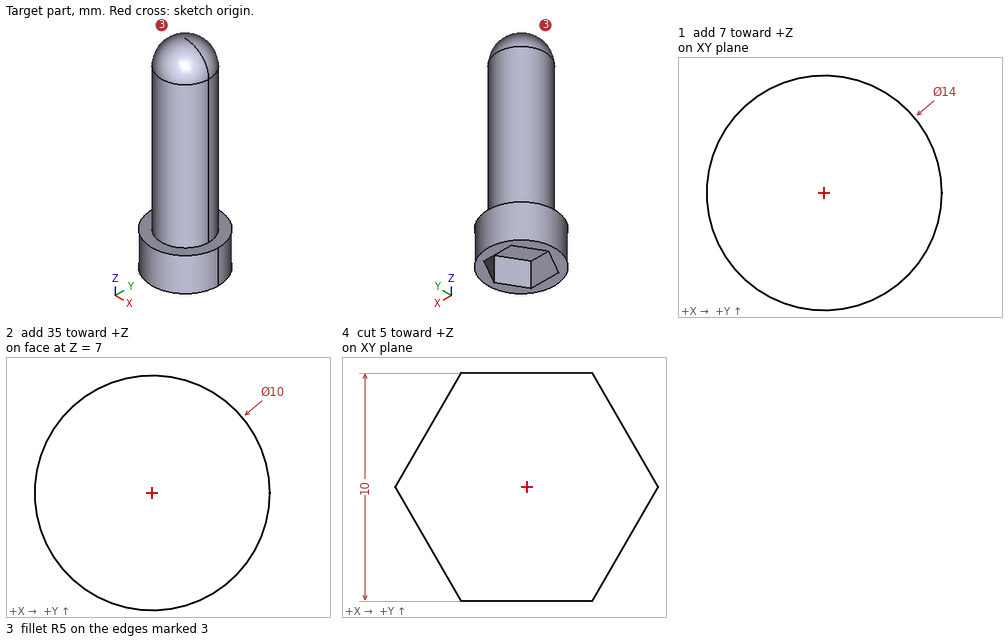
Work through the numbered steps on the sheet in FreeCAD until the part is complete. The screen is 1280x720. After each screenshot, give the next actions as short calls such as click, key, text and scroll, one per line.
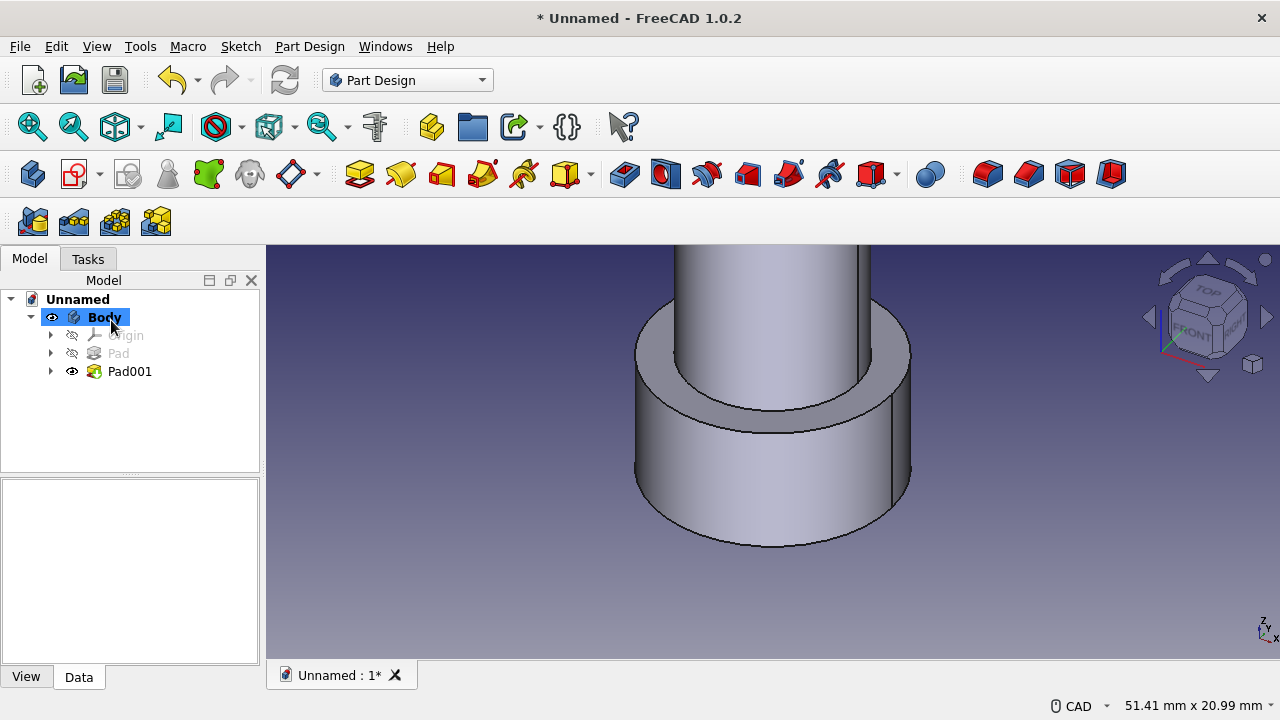
key(v)
key(f)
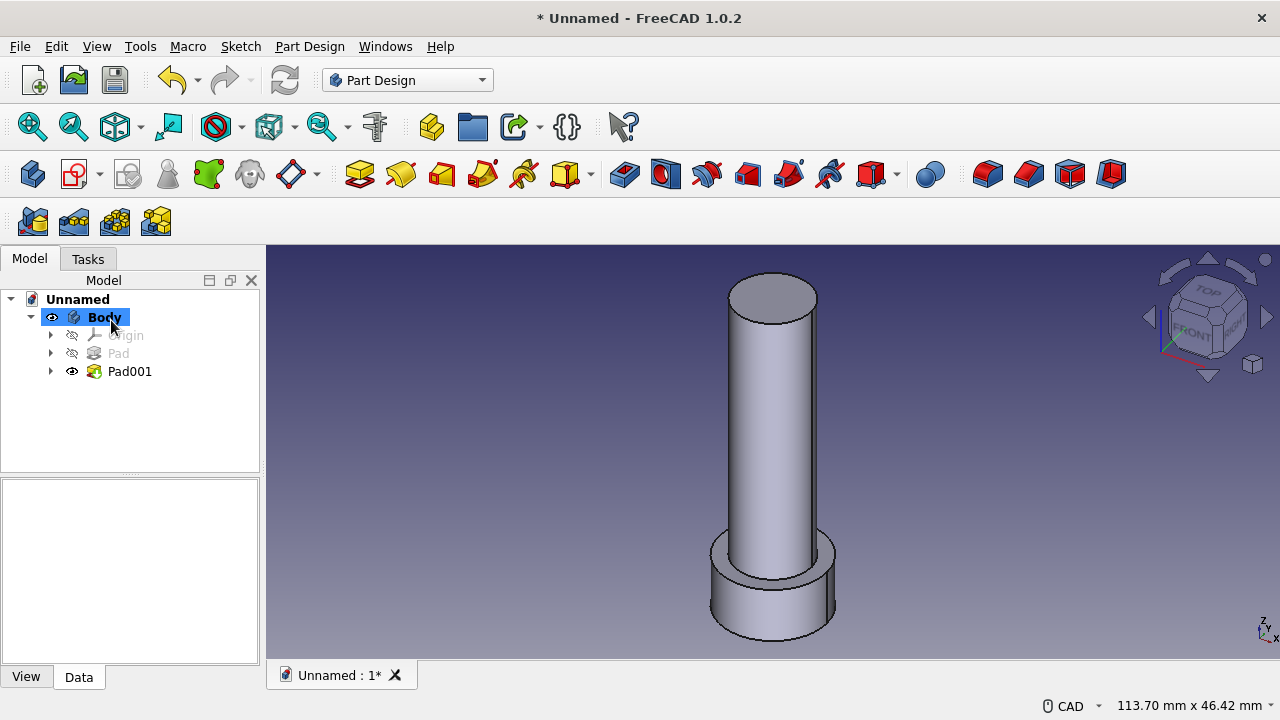
click(734, 285)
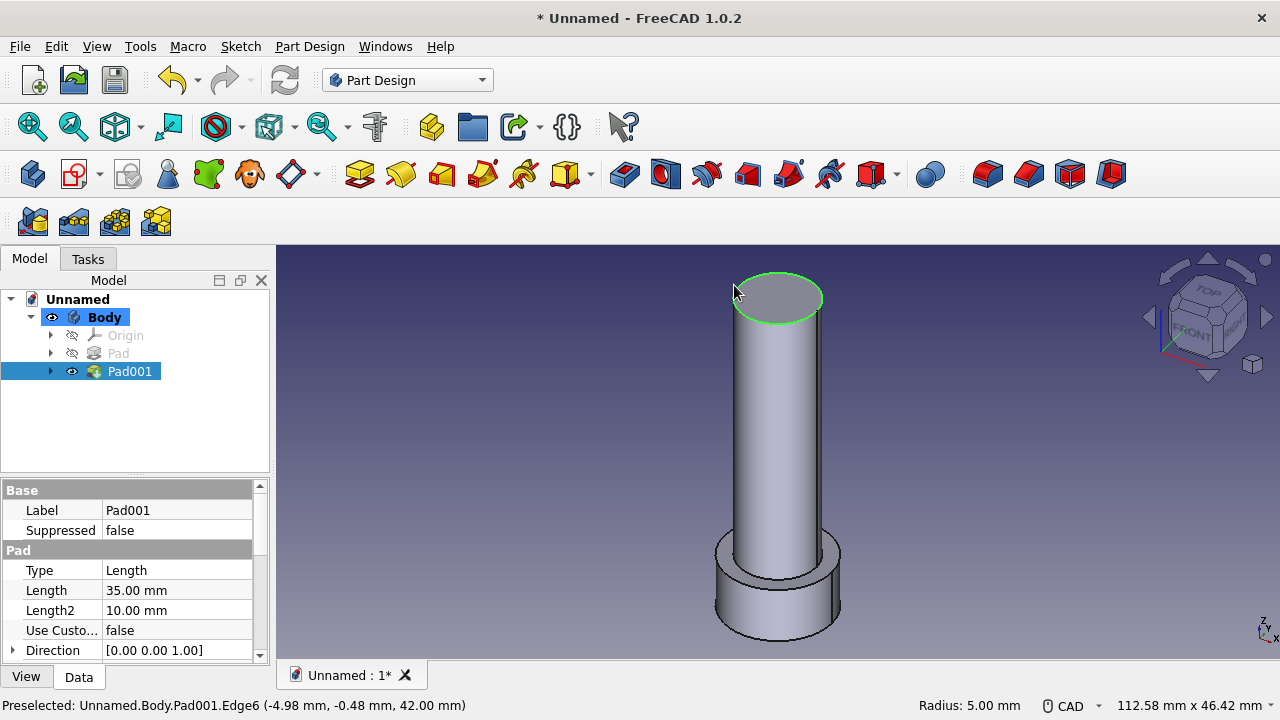
click(988, 174)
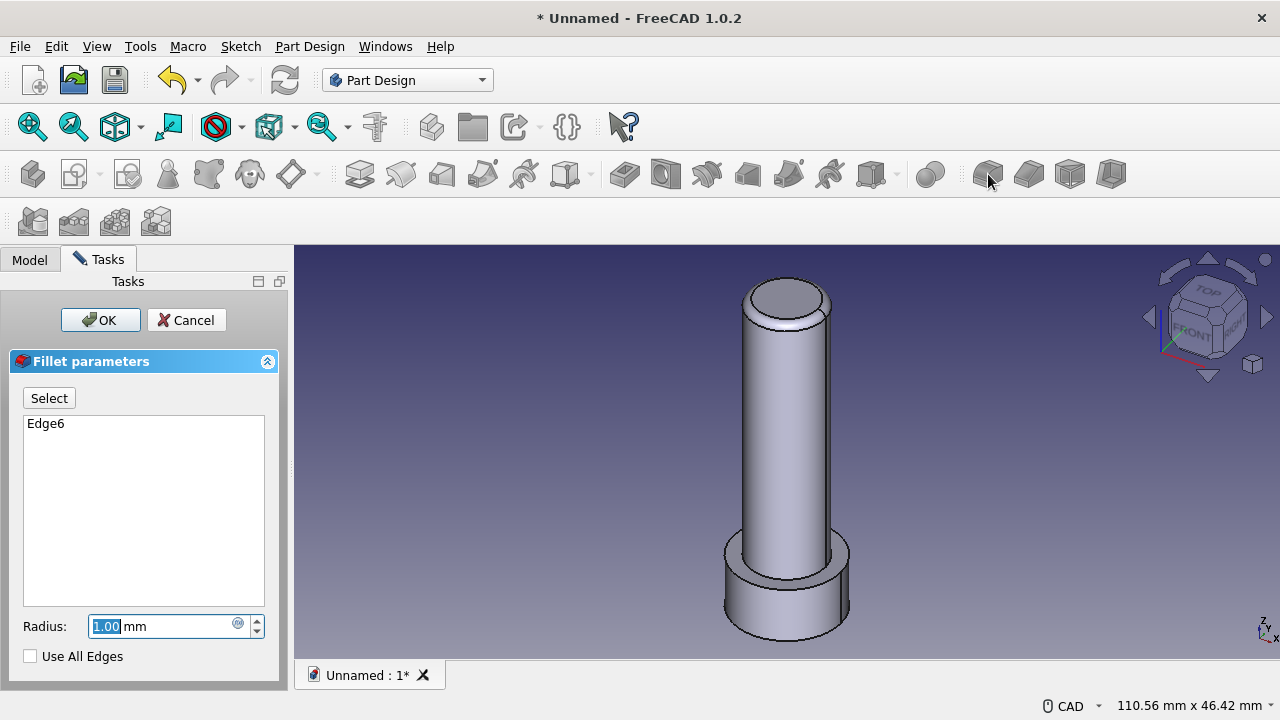
text(5)
key(Tab)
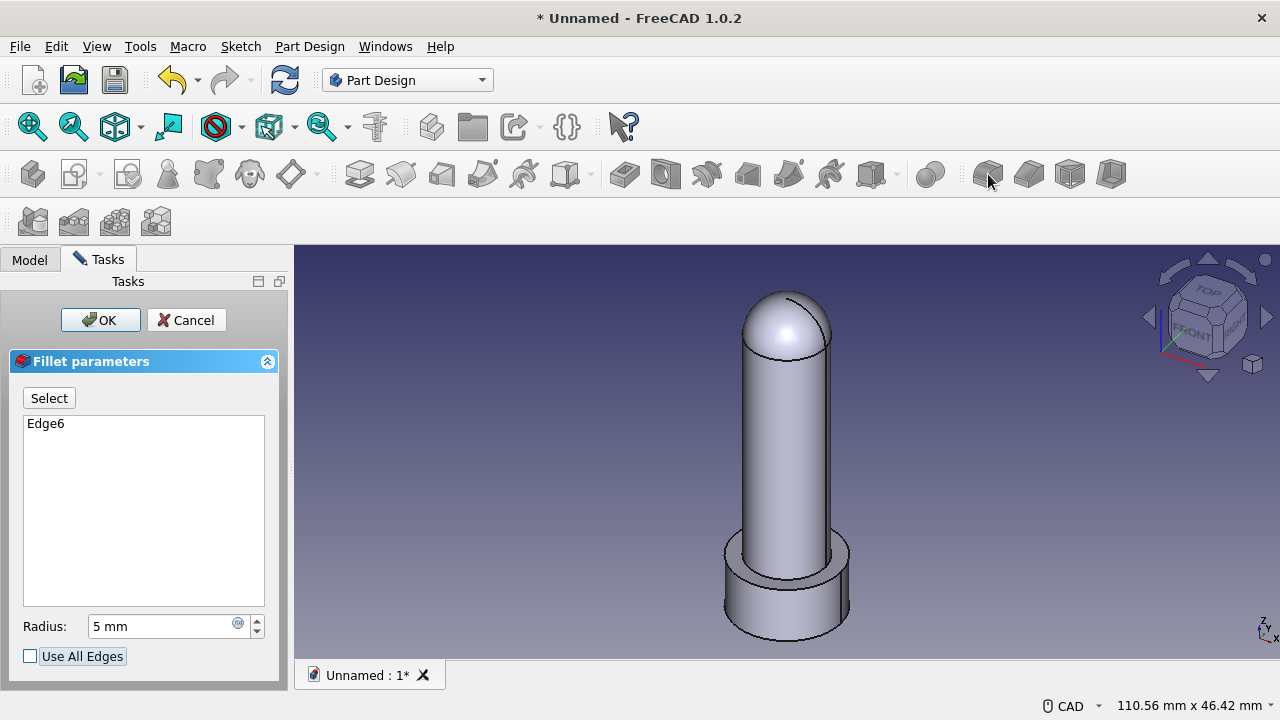
click(101, 320)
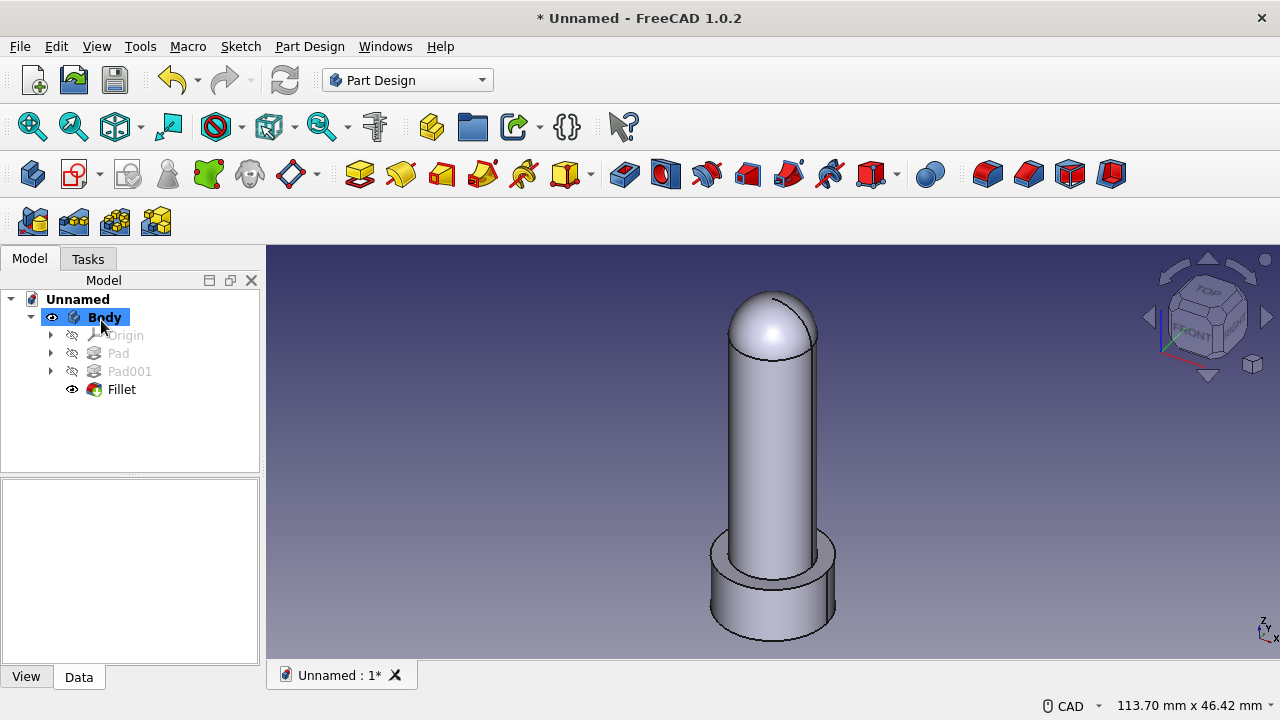
click(74, 174)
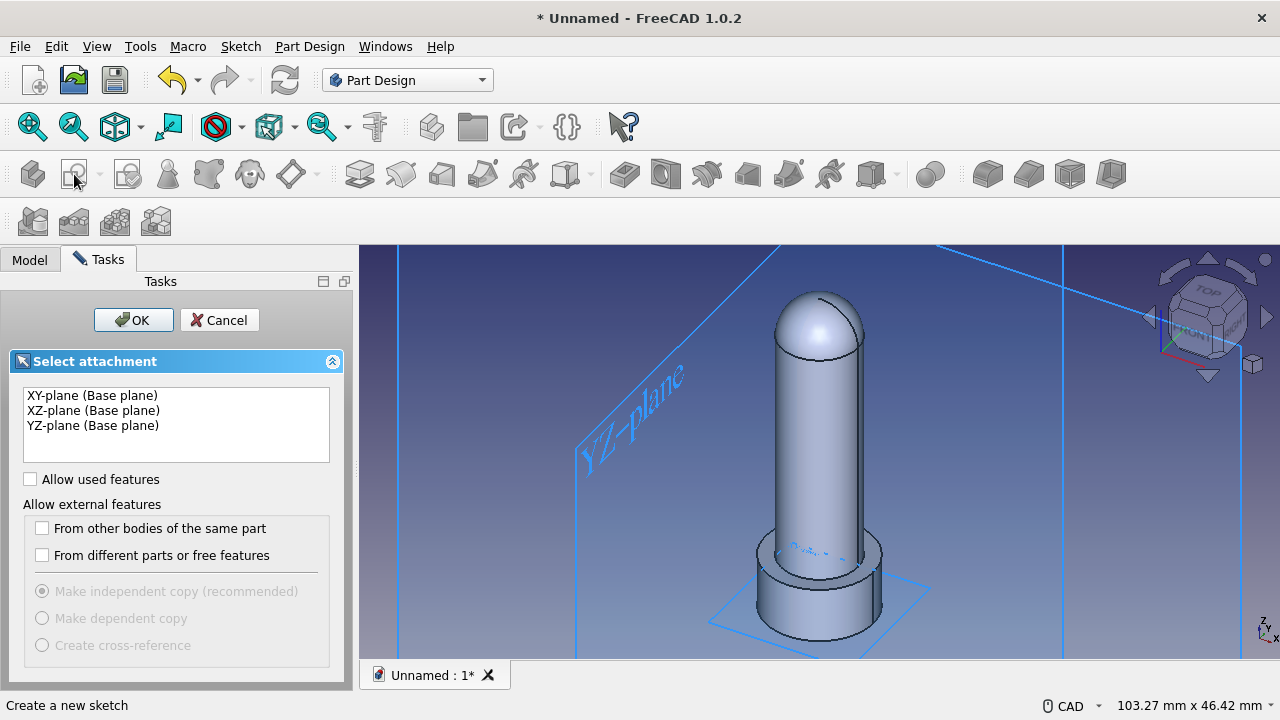
click(84, 396)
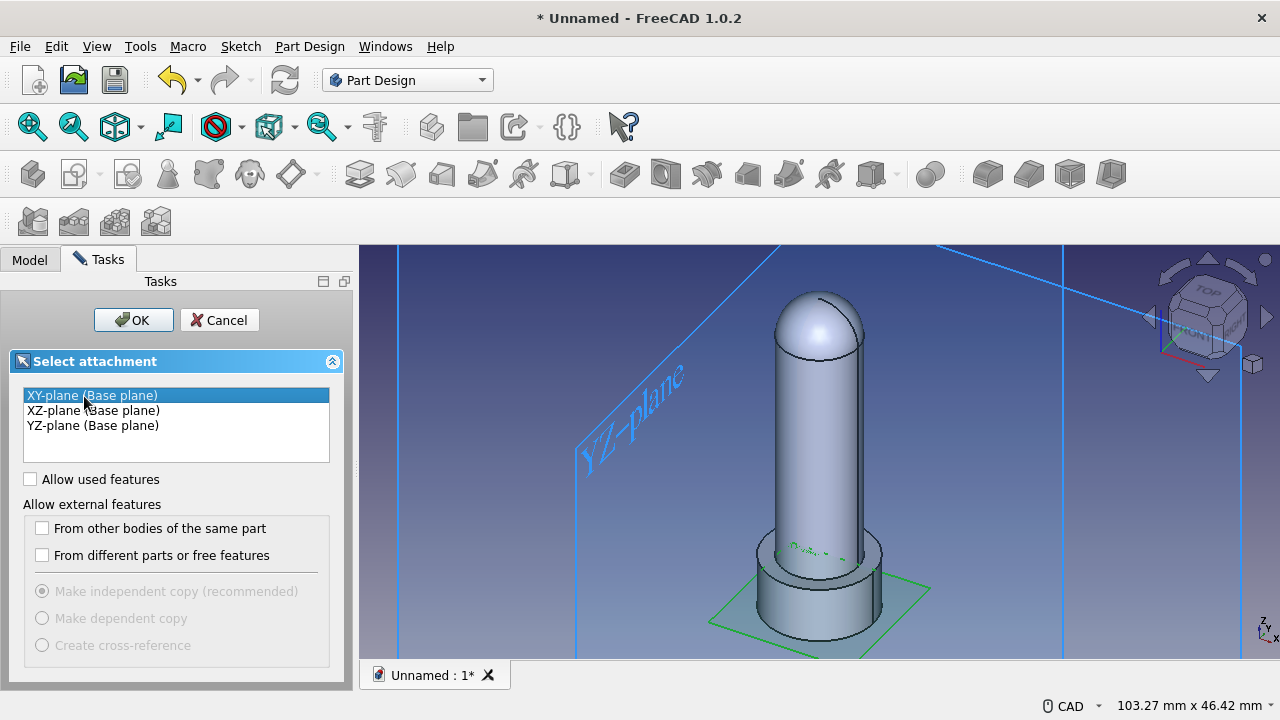
click(134, 320)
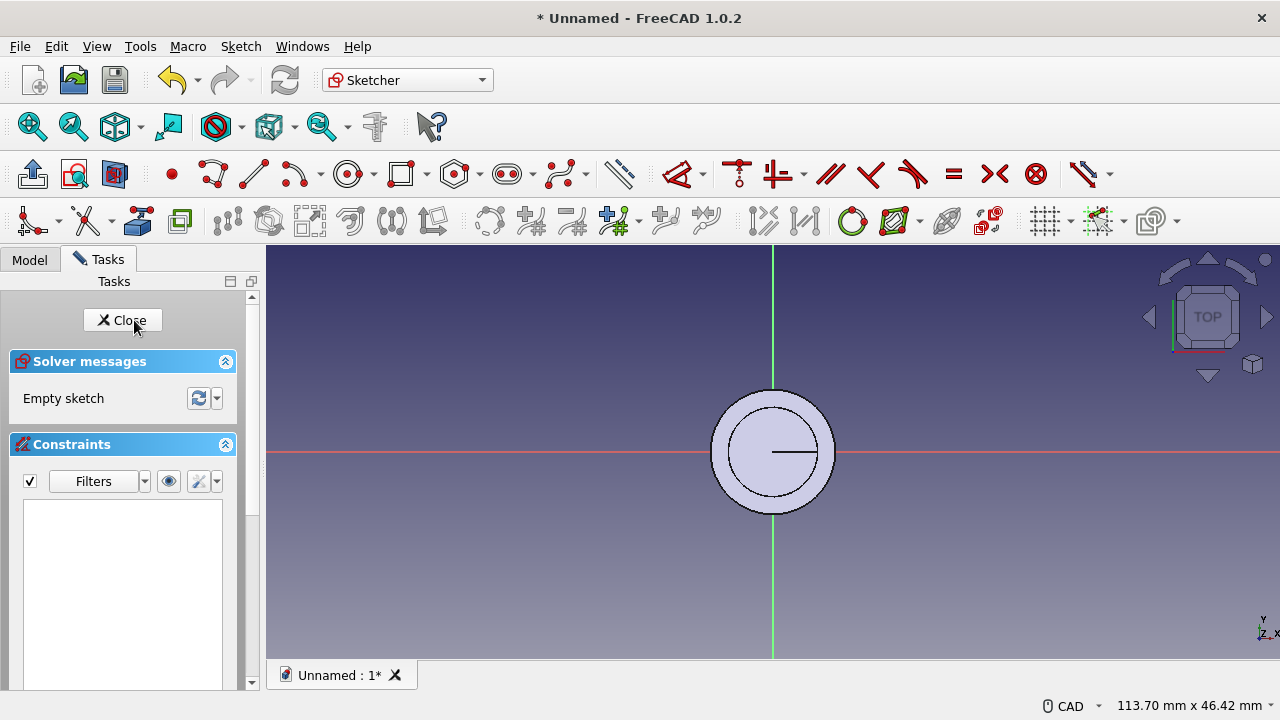
key(q)
key(s)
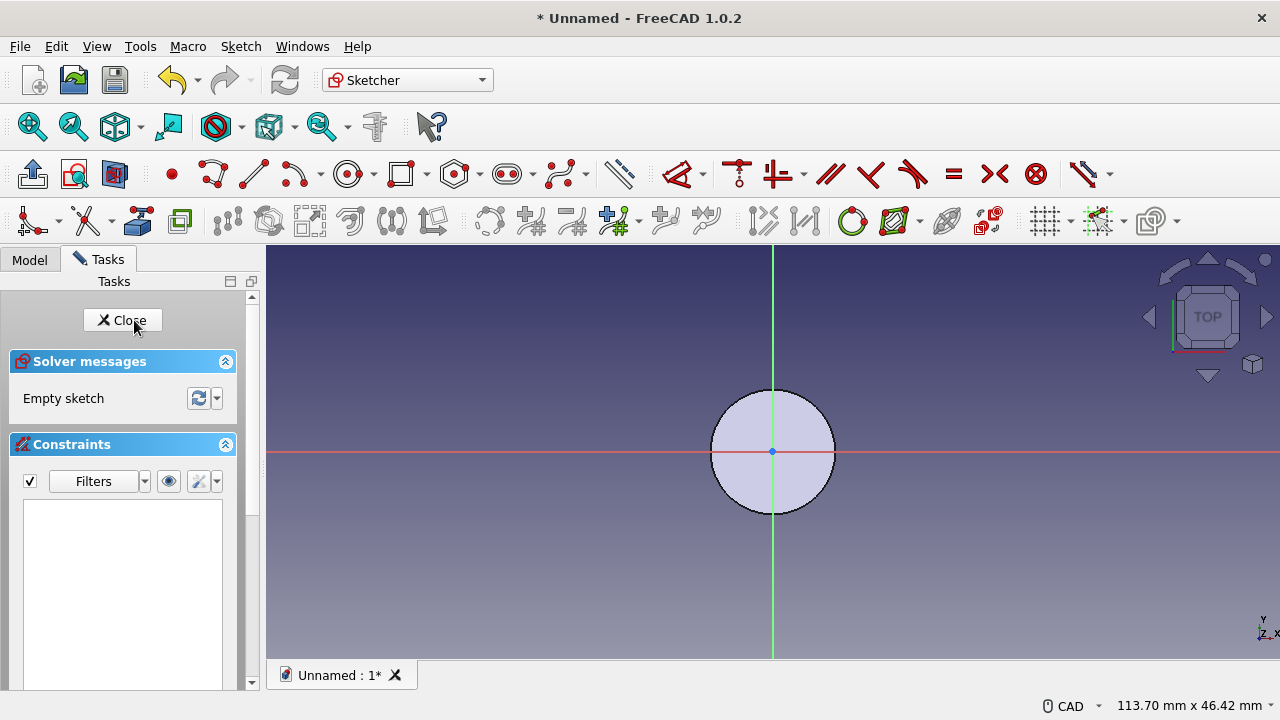
scroll(813, 452, up, 5)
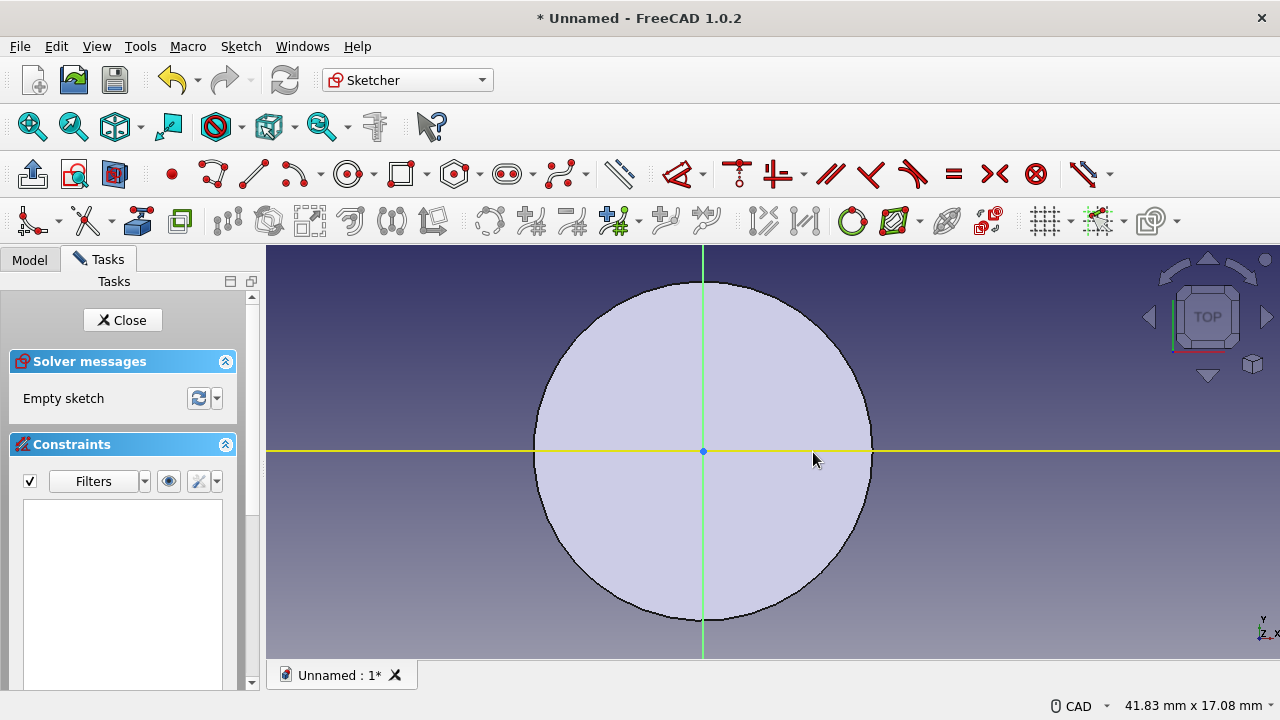
key(g)
key(p)
key(6)